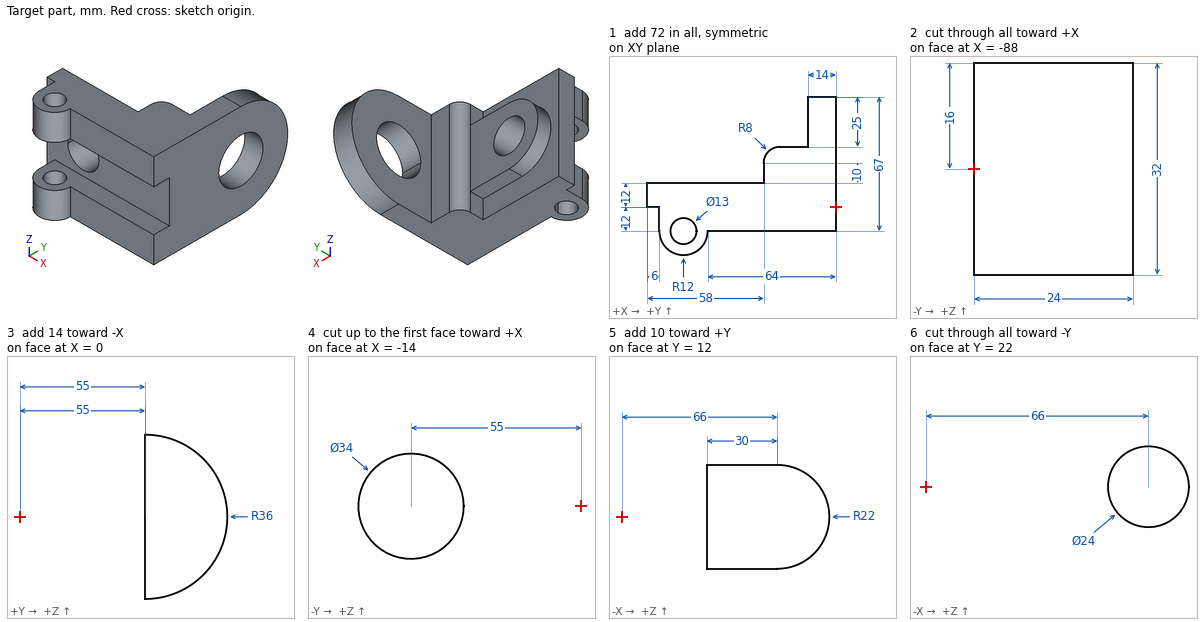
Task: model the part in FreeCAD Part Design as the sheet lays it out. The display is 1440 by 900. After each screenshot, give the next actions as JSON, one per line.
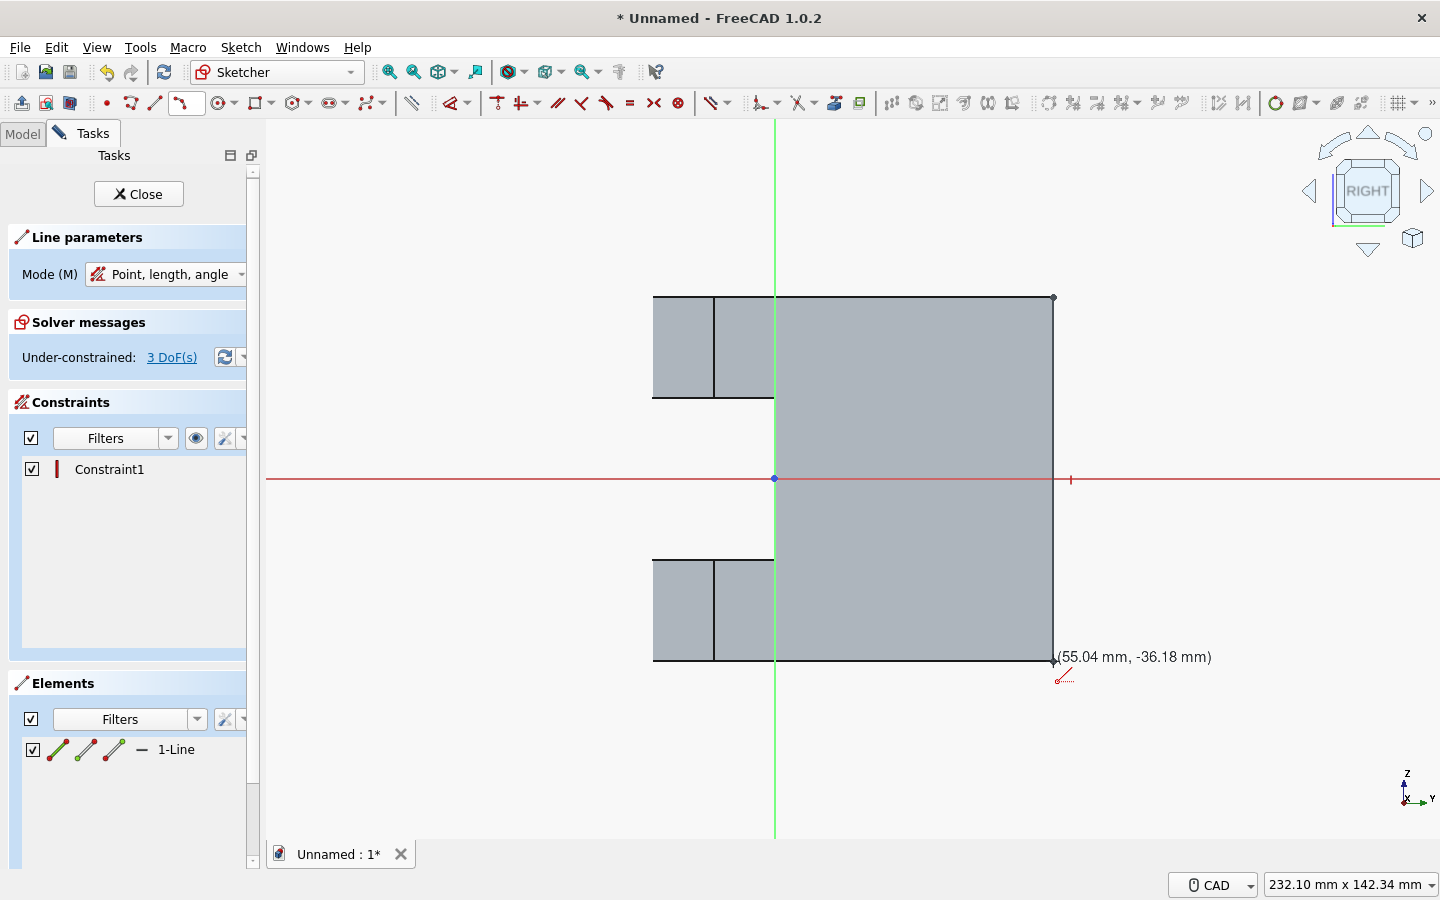
{"action": "left_click", "coordinate": [180, 104]}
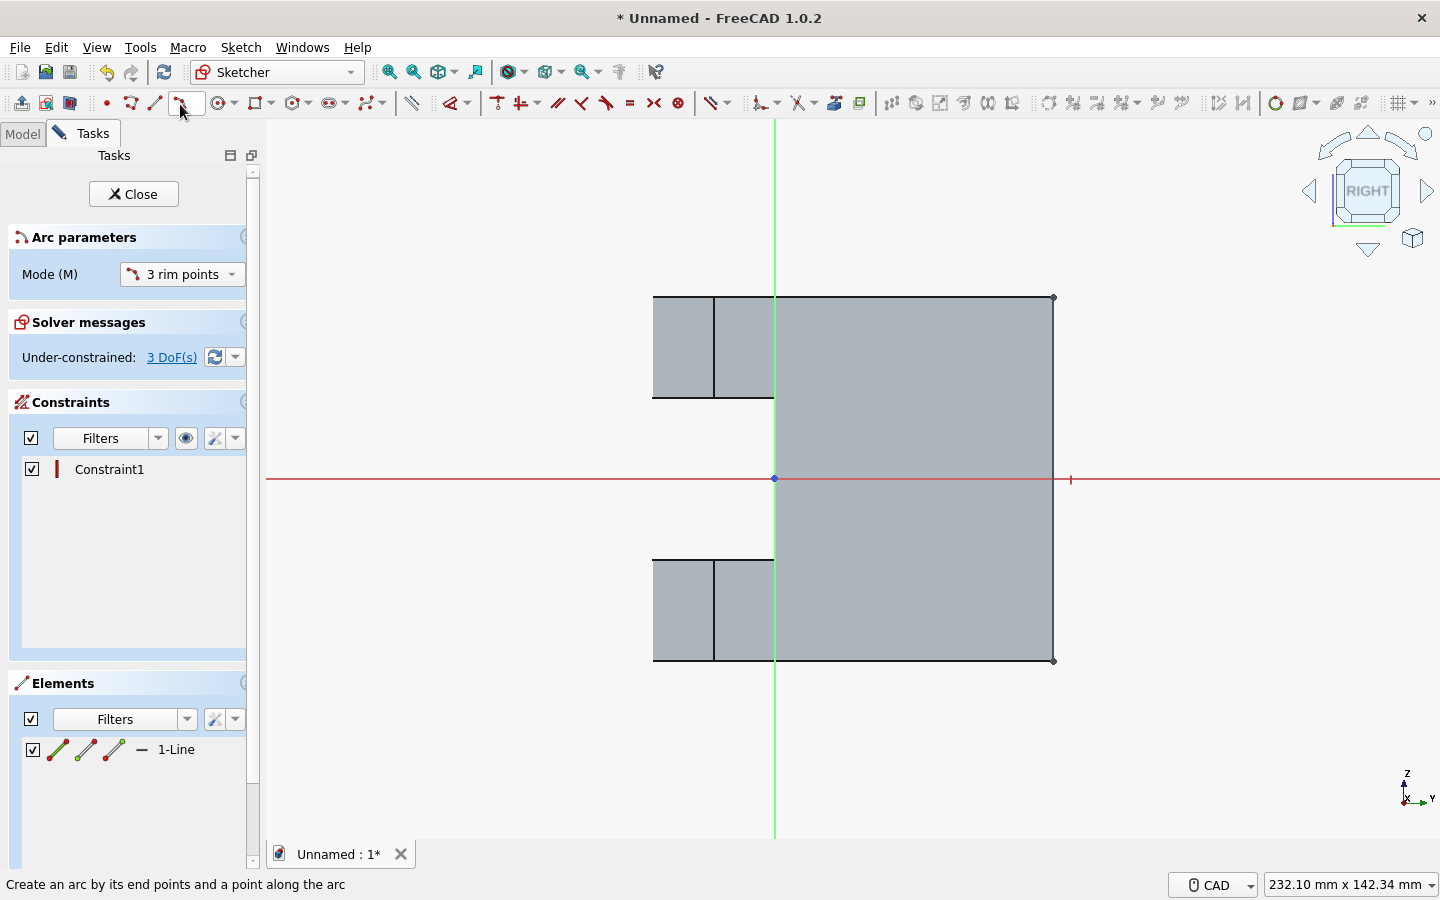
{"action": "left_click", "coordinate": [1053, 662]}
{"action": "left_click", "coordinate": [1053, 298]}
{"action": "left_click", "coordinate": [1226, 535]}
{"action": "key", "text": "Escape"}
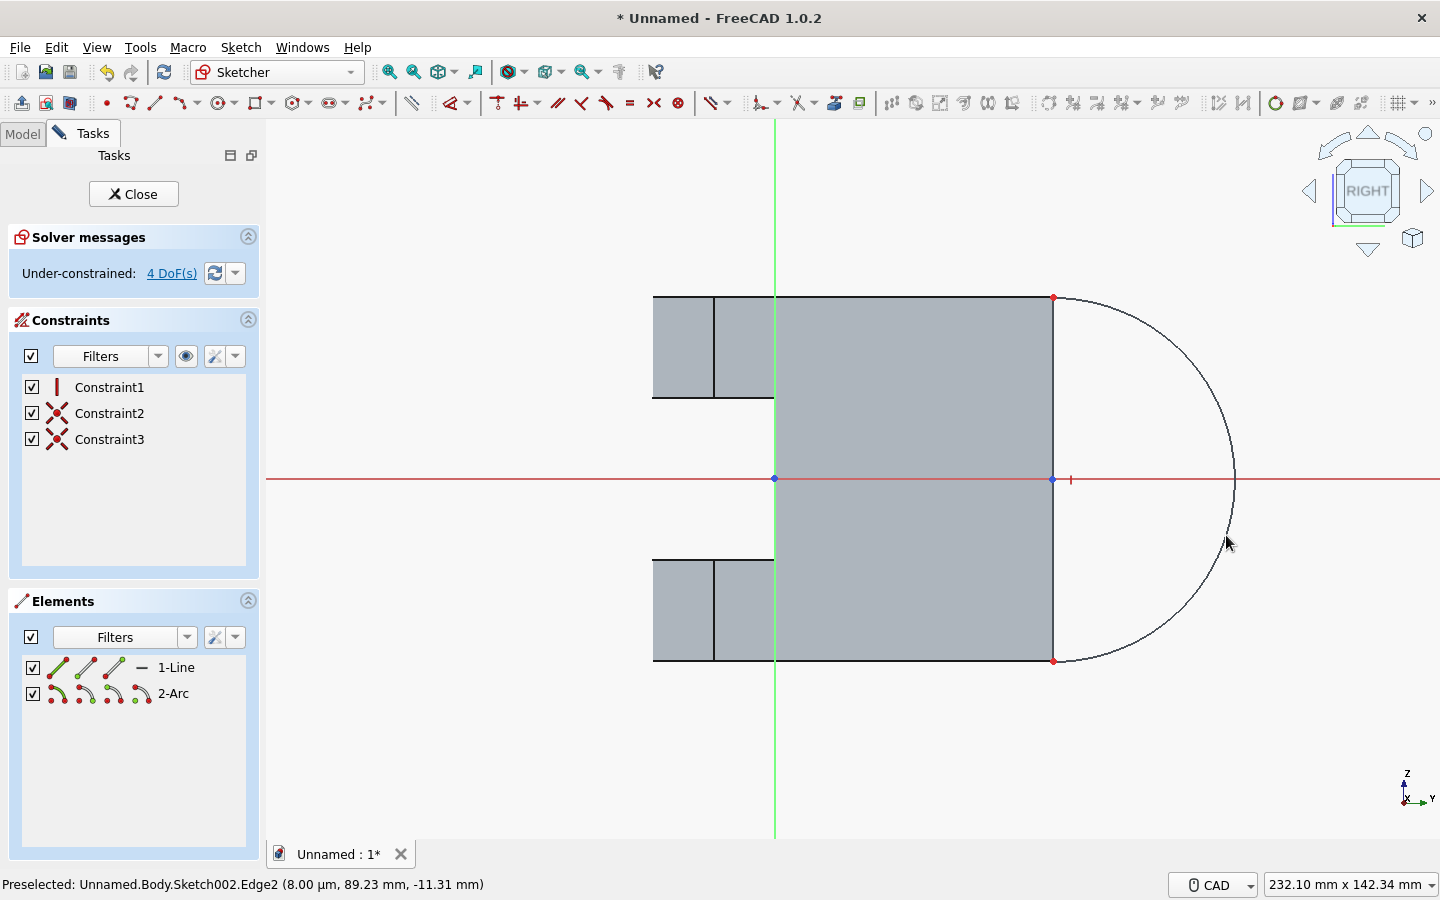
{"action": "left_click", "coordinate": [1053, 480]}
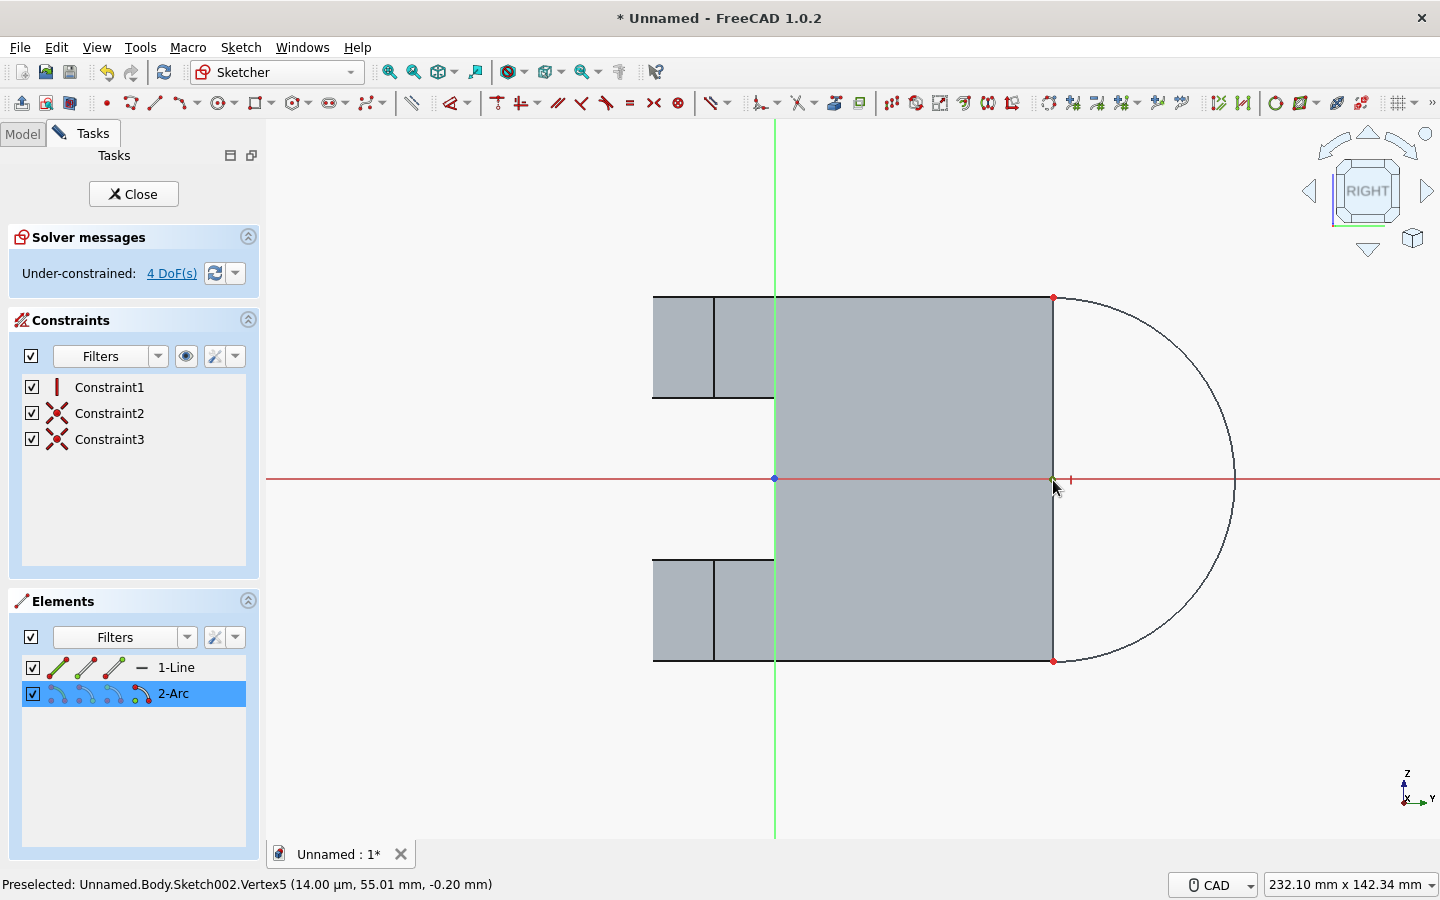
{"action": "left_click", "coordinate": [364, 479]}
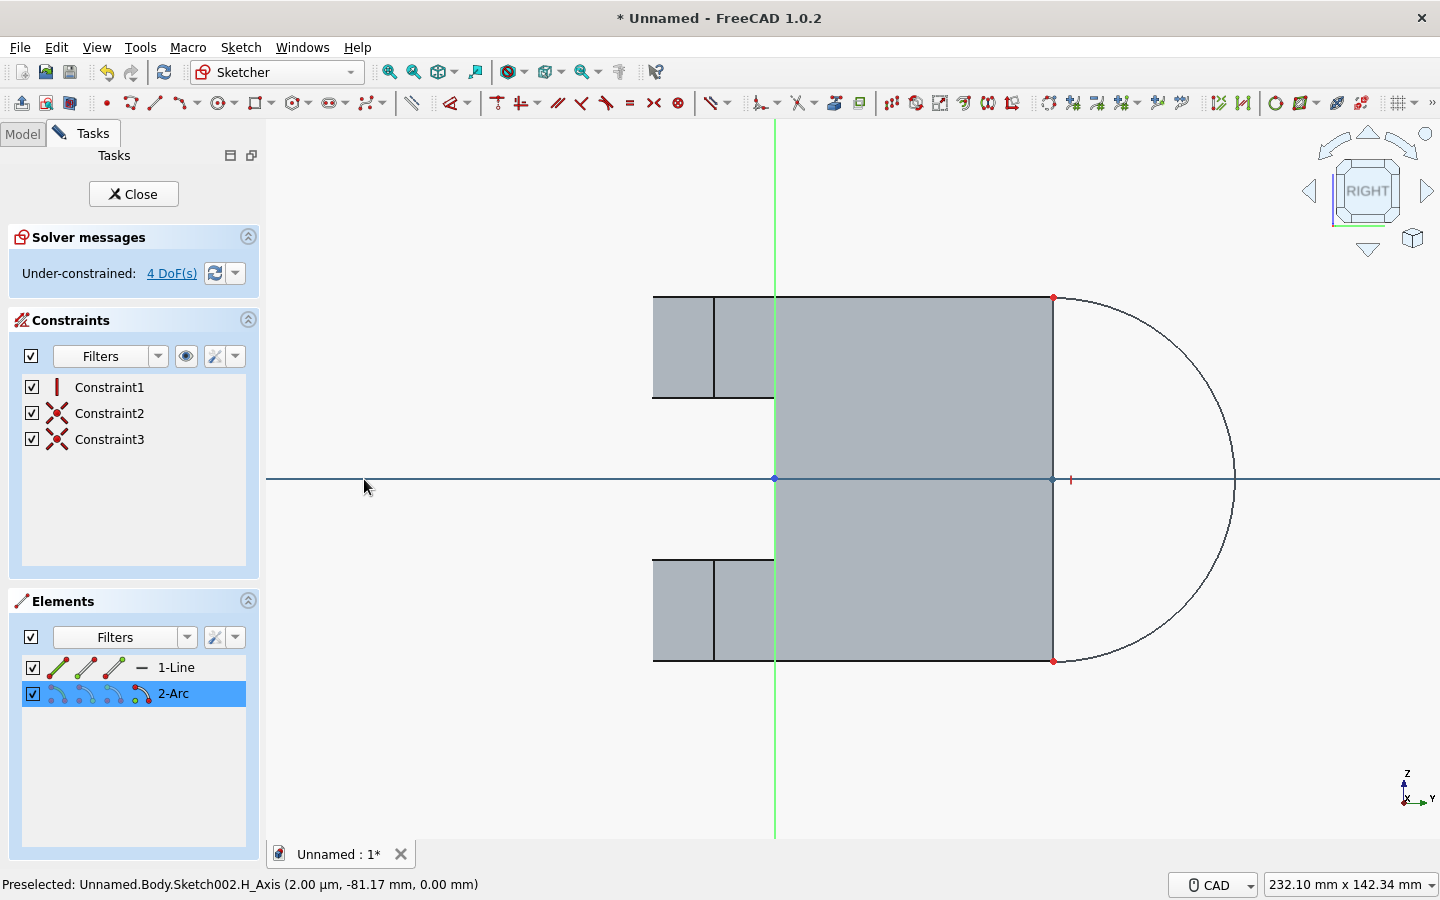
{"action": "left_click", "coordinate": [498, 104]}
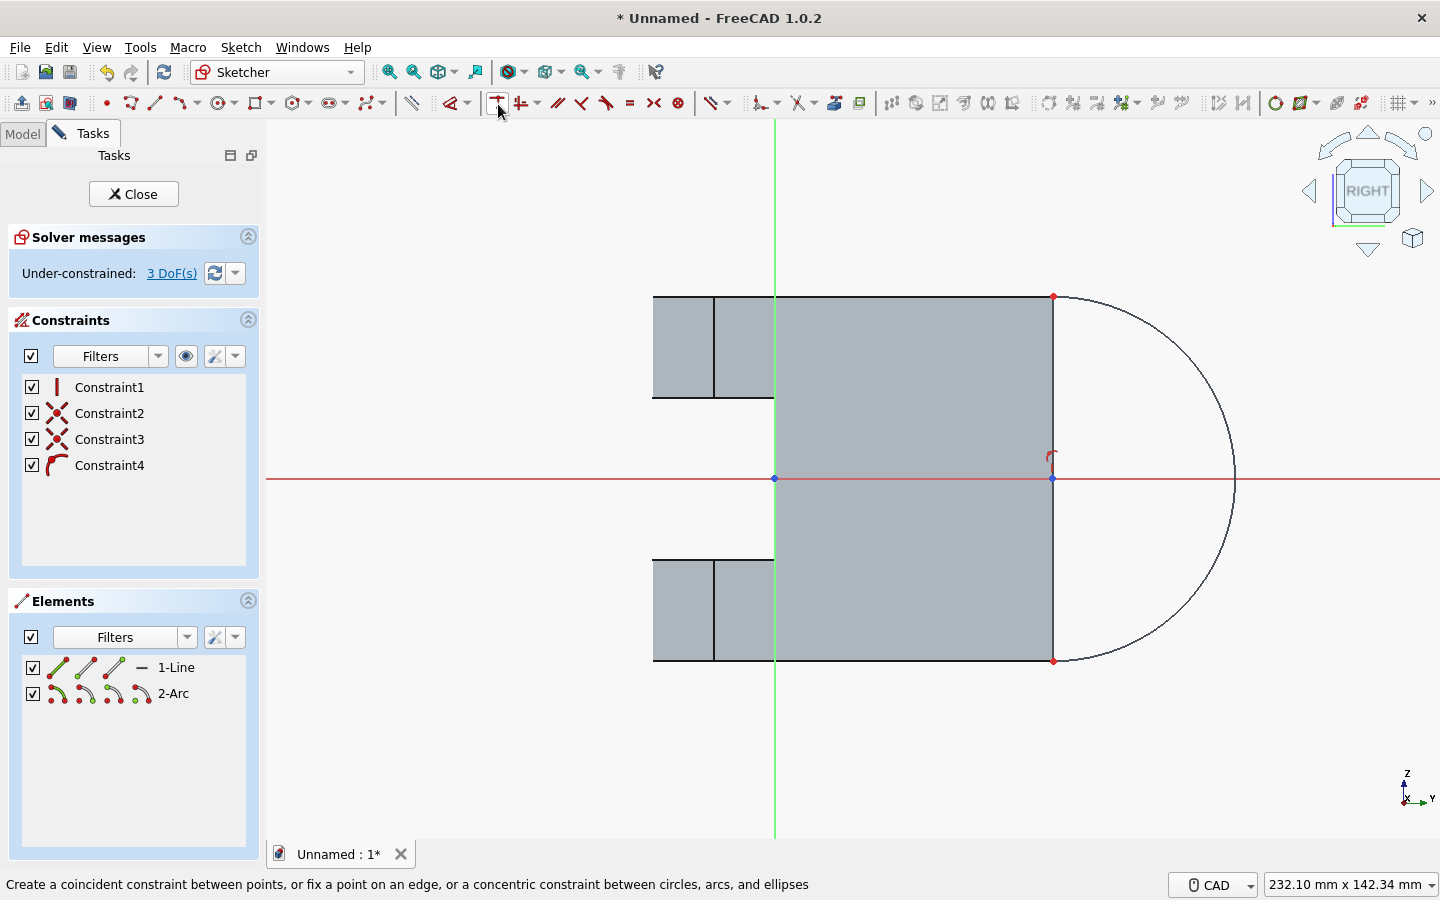
{"action": "left_click", "coordinate": [450, 104]}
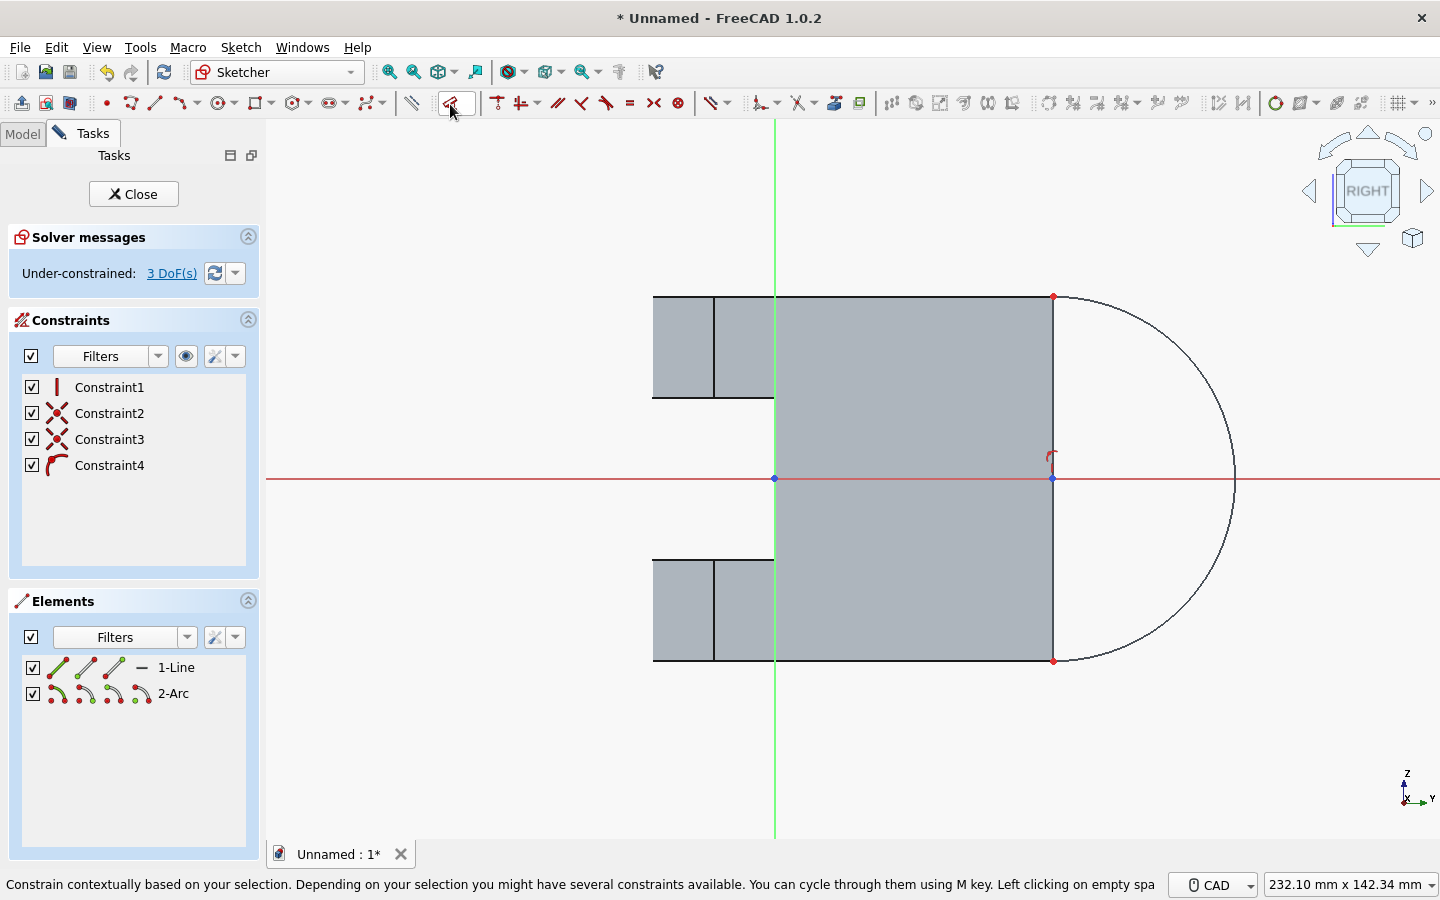
{"action": "left_click", "coordinate": [1200, 586]}
{"action": "left_click", "coordinate": [1226, 605]}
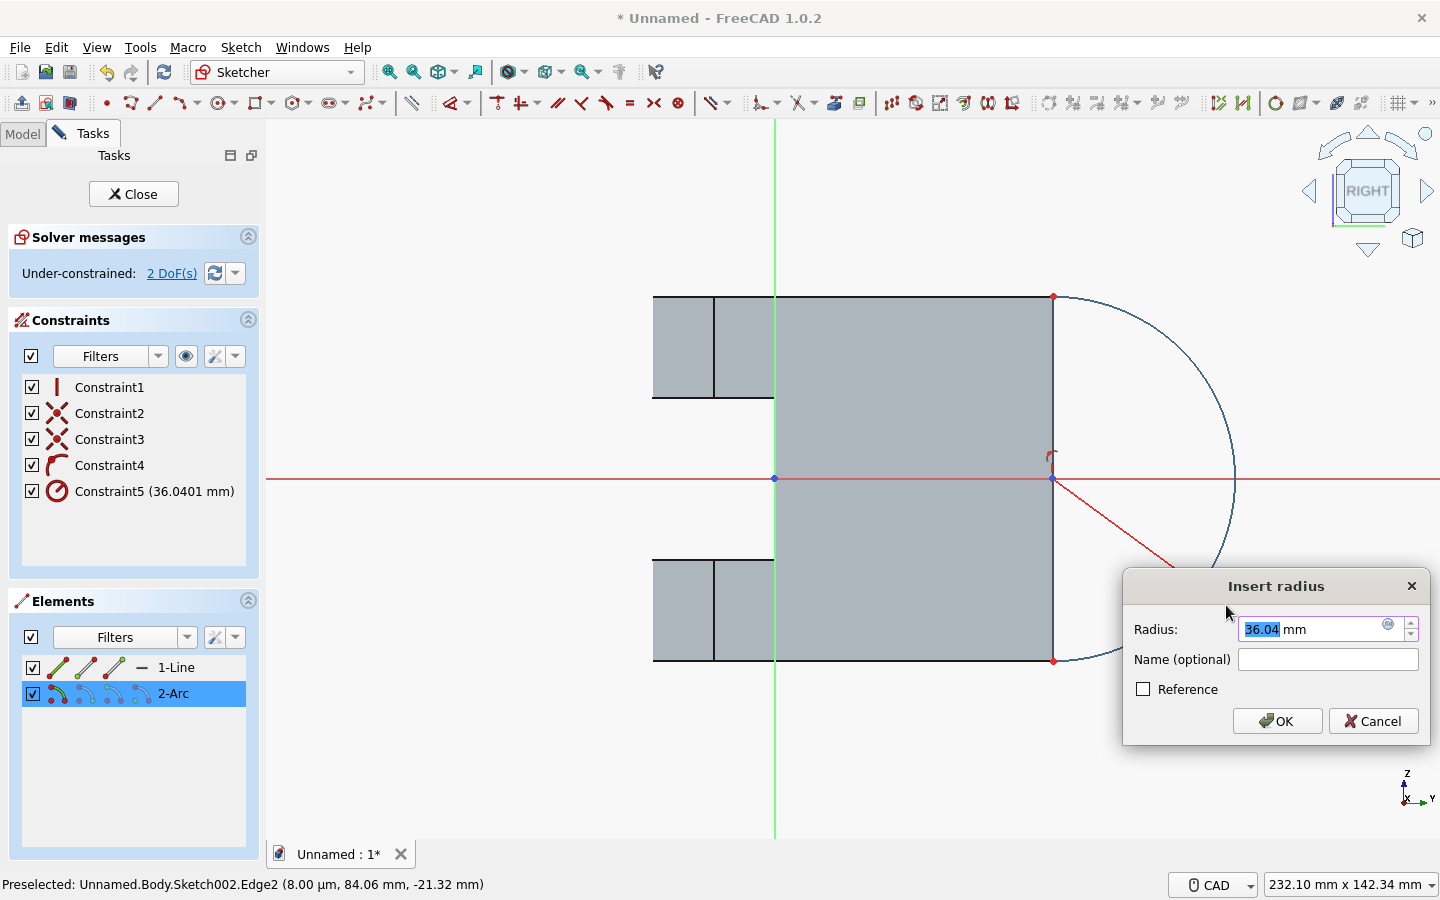
{"action": "type", "text": "36"}
{"action": "key", "text": "Return"}